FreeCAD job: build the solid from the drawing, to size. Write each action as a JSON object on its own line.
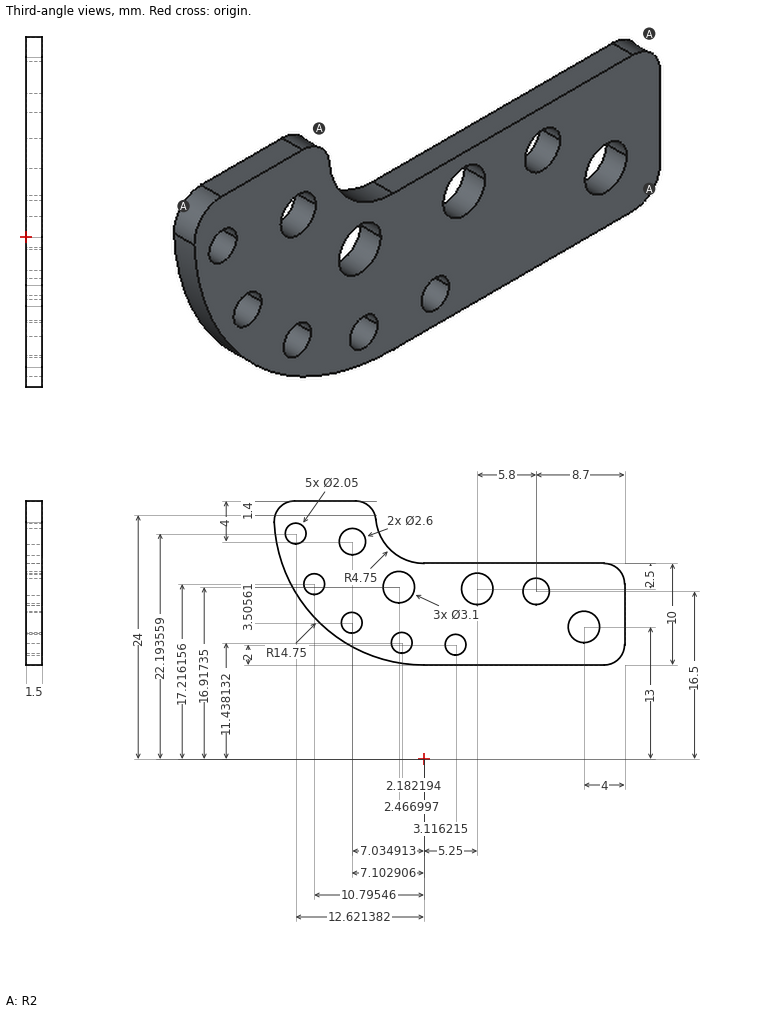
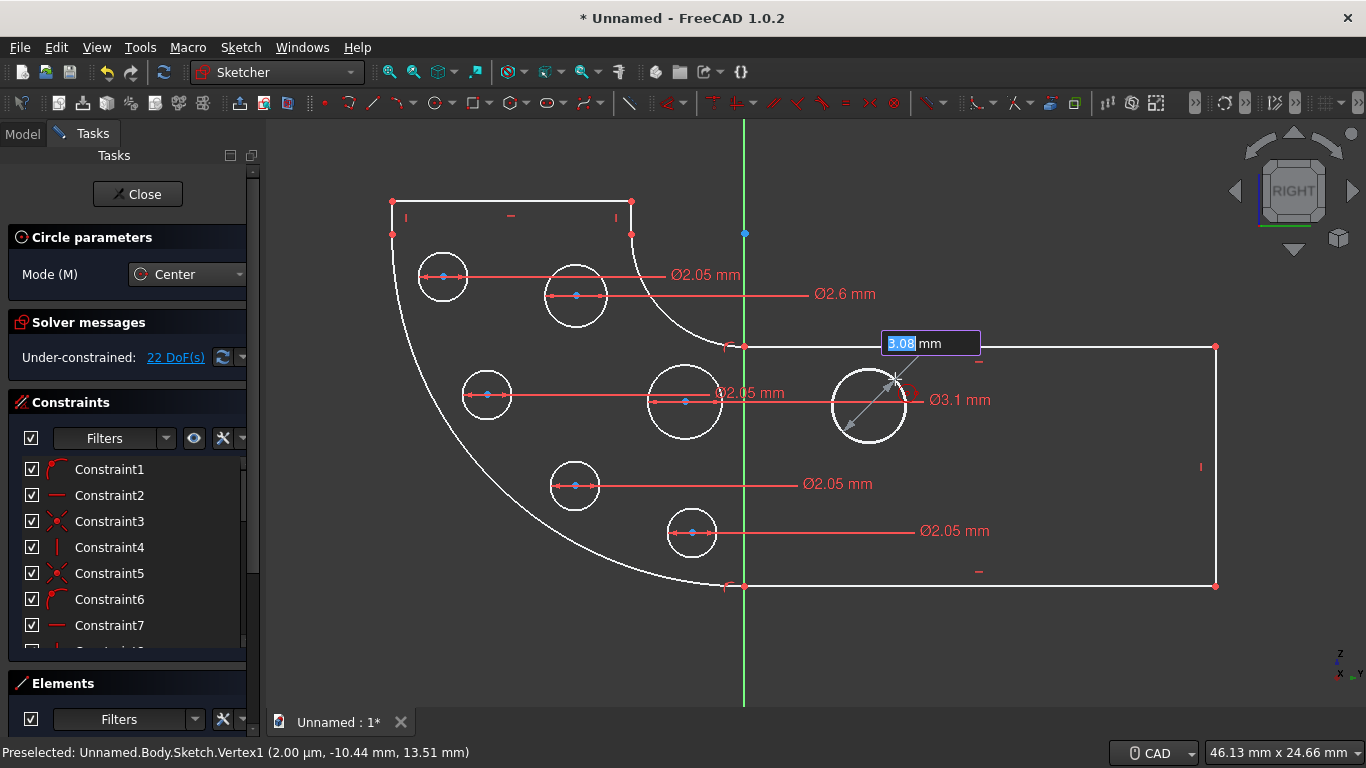
{"action": "type", "text": "3.1"}
{"action": "key", "text": "Return"}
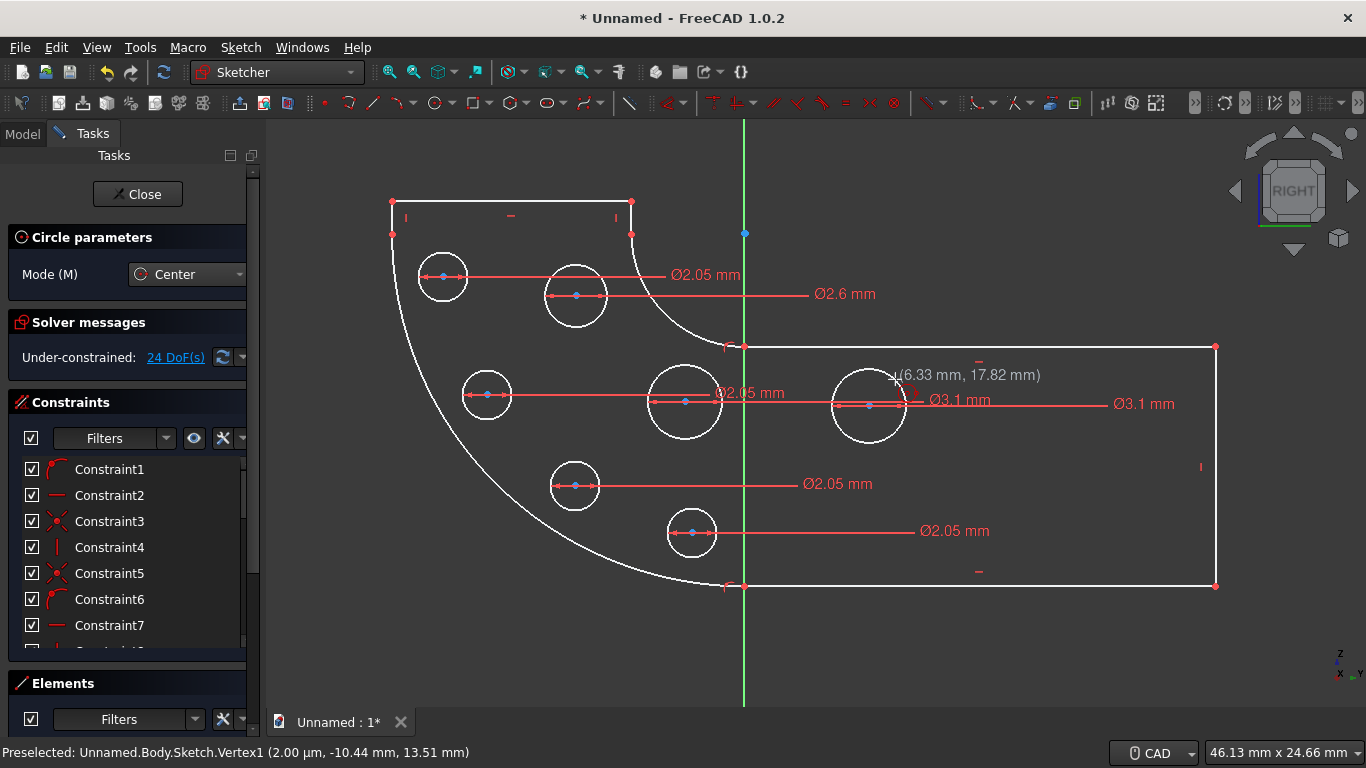
{"action": "left_click", "coordinate": [818, 537]}
{"action": "mouse_move", "coordinate": [836, 519]}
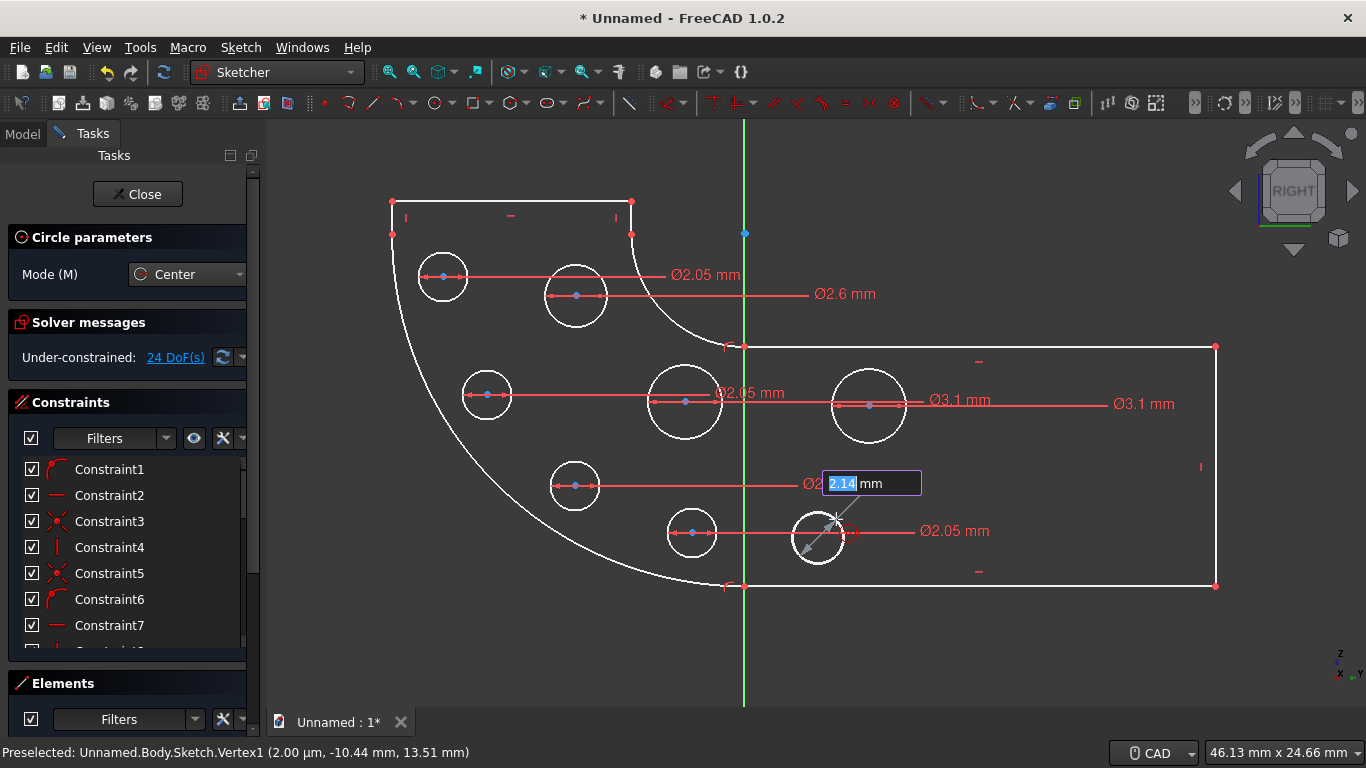
{"action": "type", "text": "2.05"}
{"action": "key", "text": "Return"}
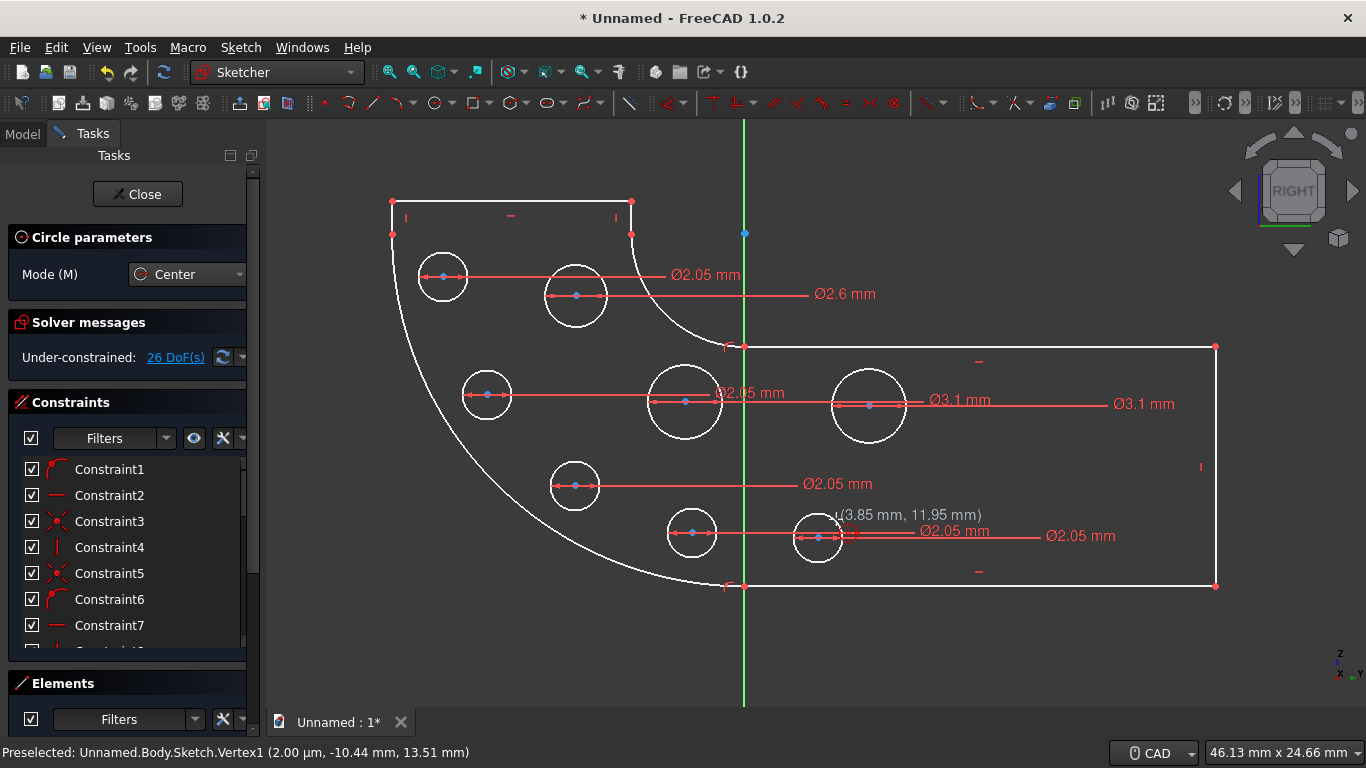
{"action": "left_click", "coordinate": [1008, 411]}
{"action": "mouse_move", "coordinate": [1030, 390]}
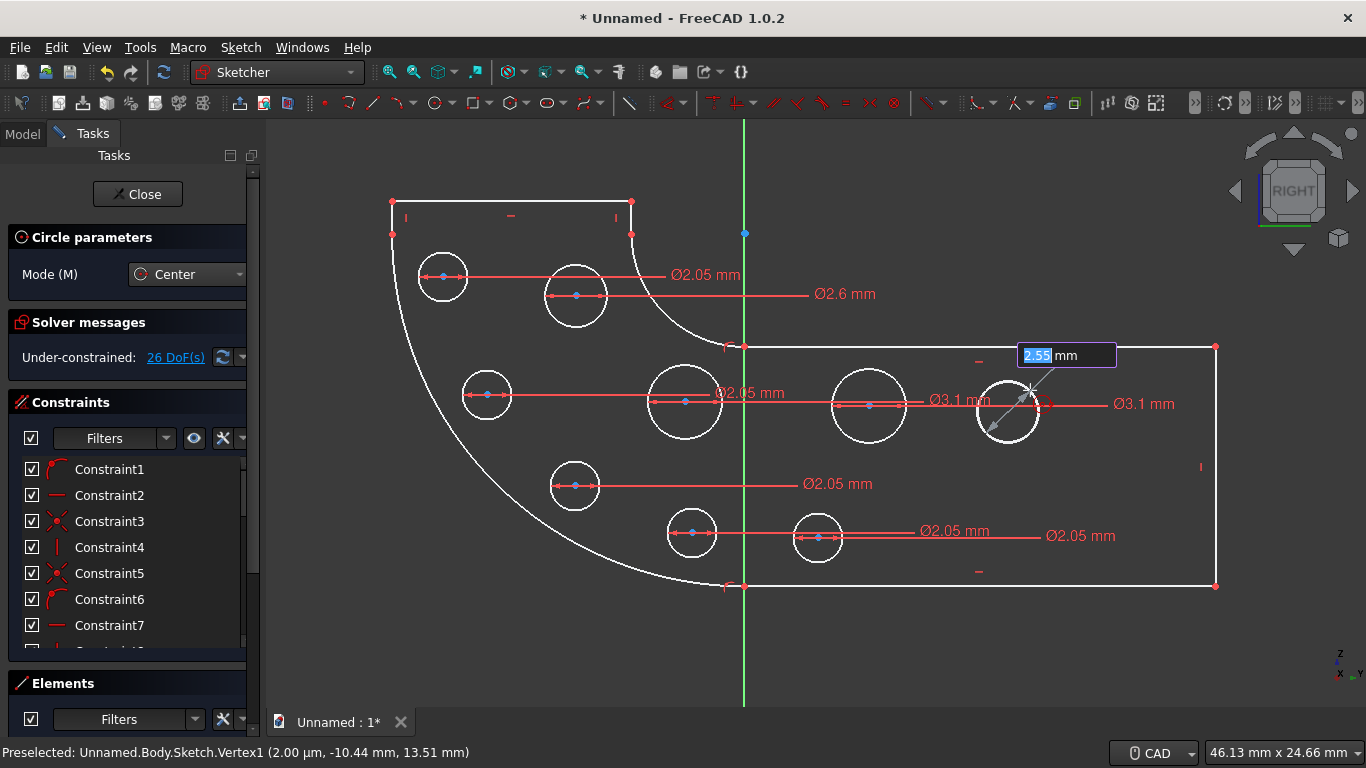
{"action": "type", "text": "2.6"}
{"action": "key", "text": "Return"}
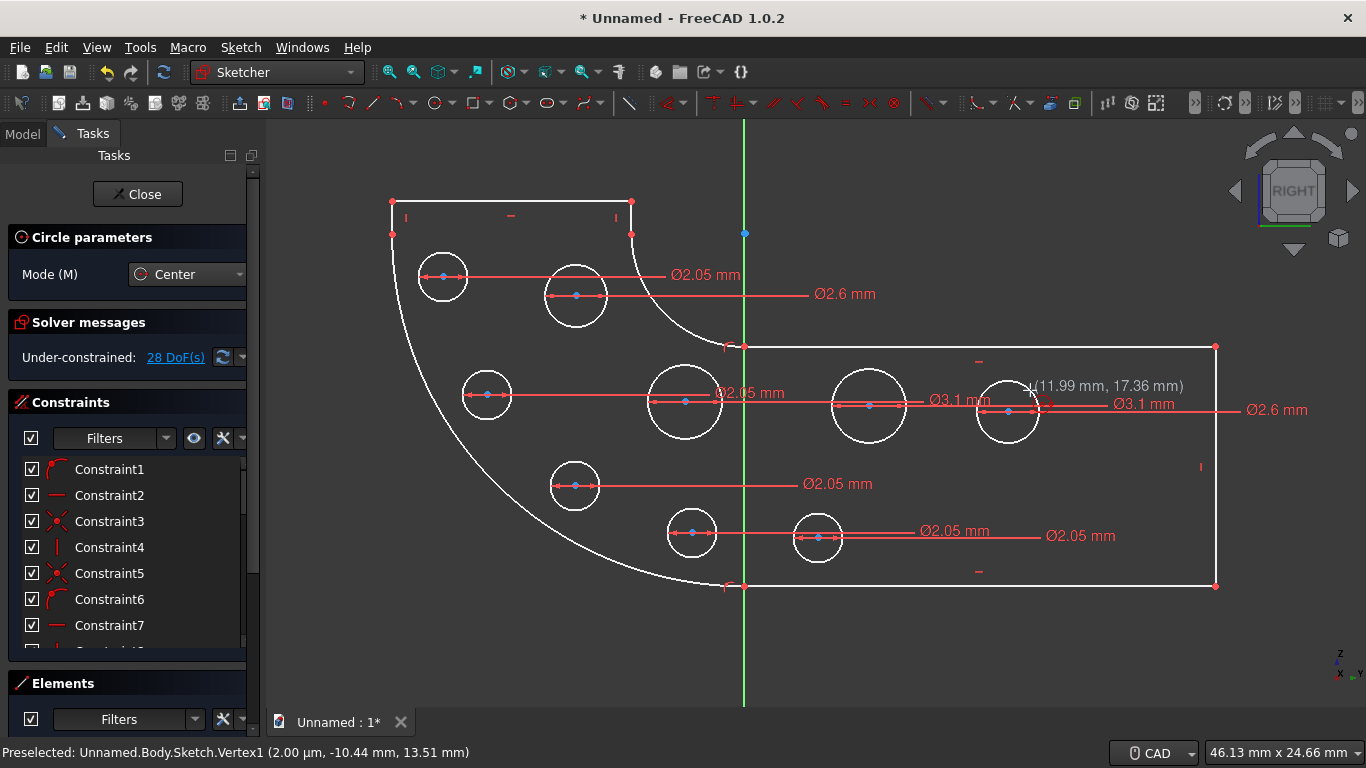
{"action": "left_click", "coordinate": [1120, 495]}
{"action": "mouse_move", "coordinate": [1146, 469]}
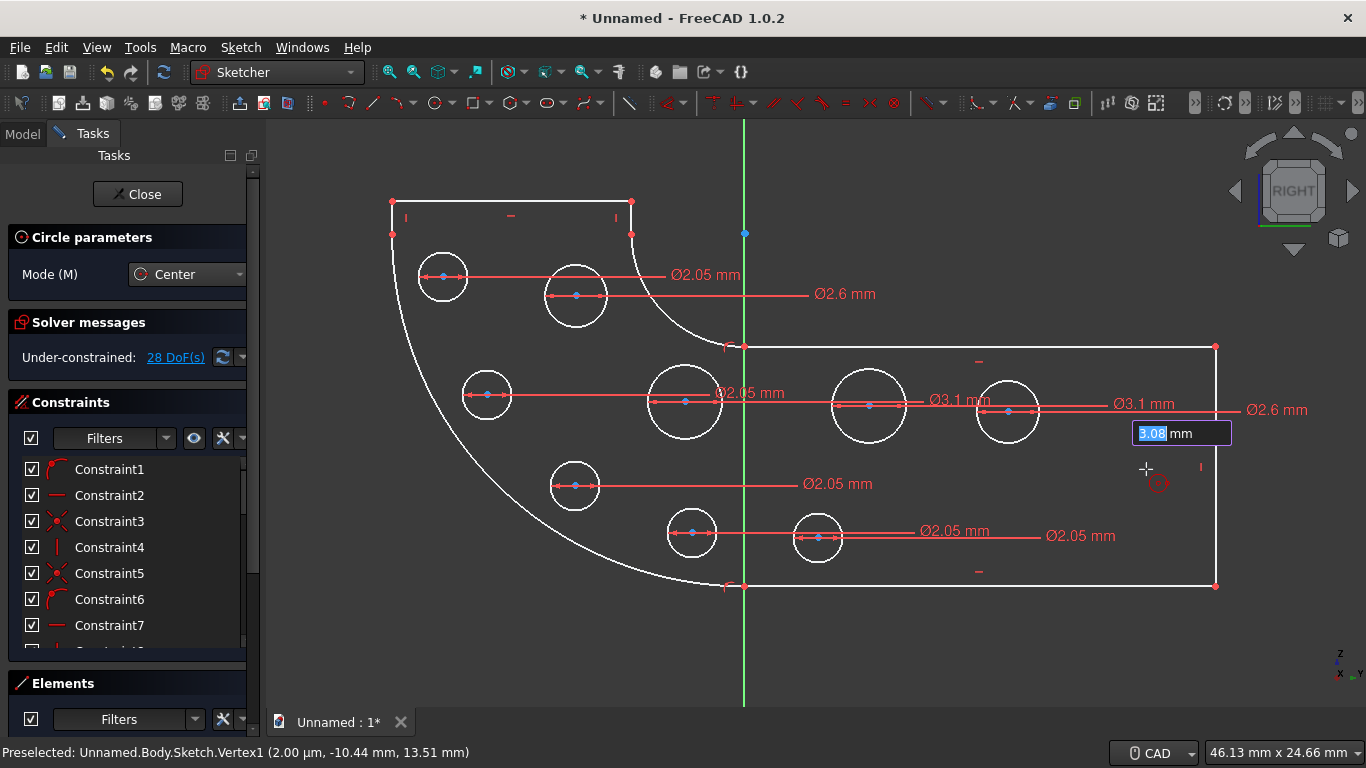
{"action": "type", "text": "3.1"}
{"action": "key", "text": "Return"}
{"action": "key", "text": "Escape"}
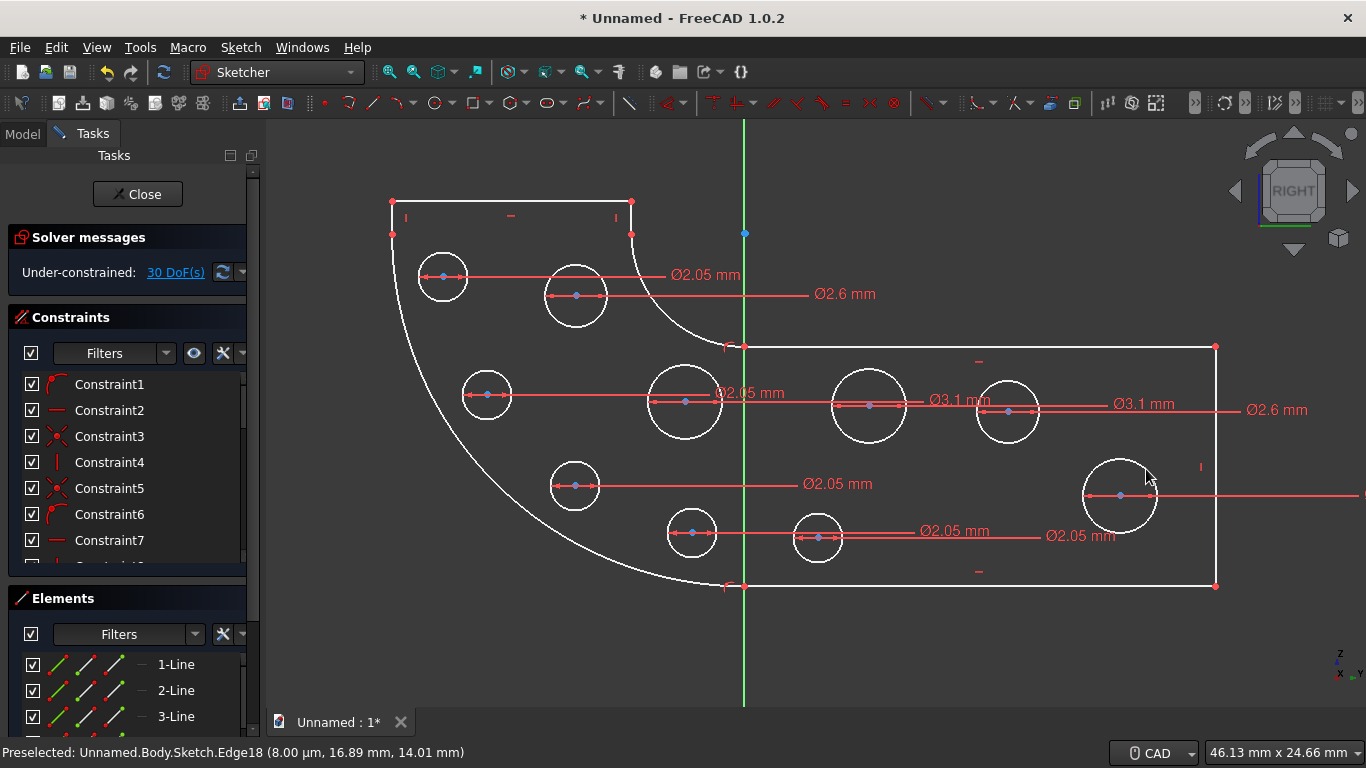
{"action": "left_click", "coordinate": [886, 586]}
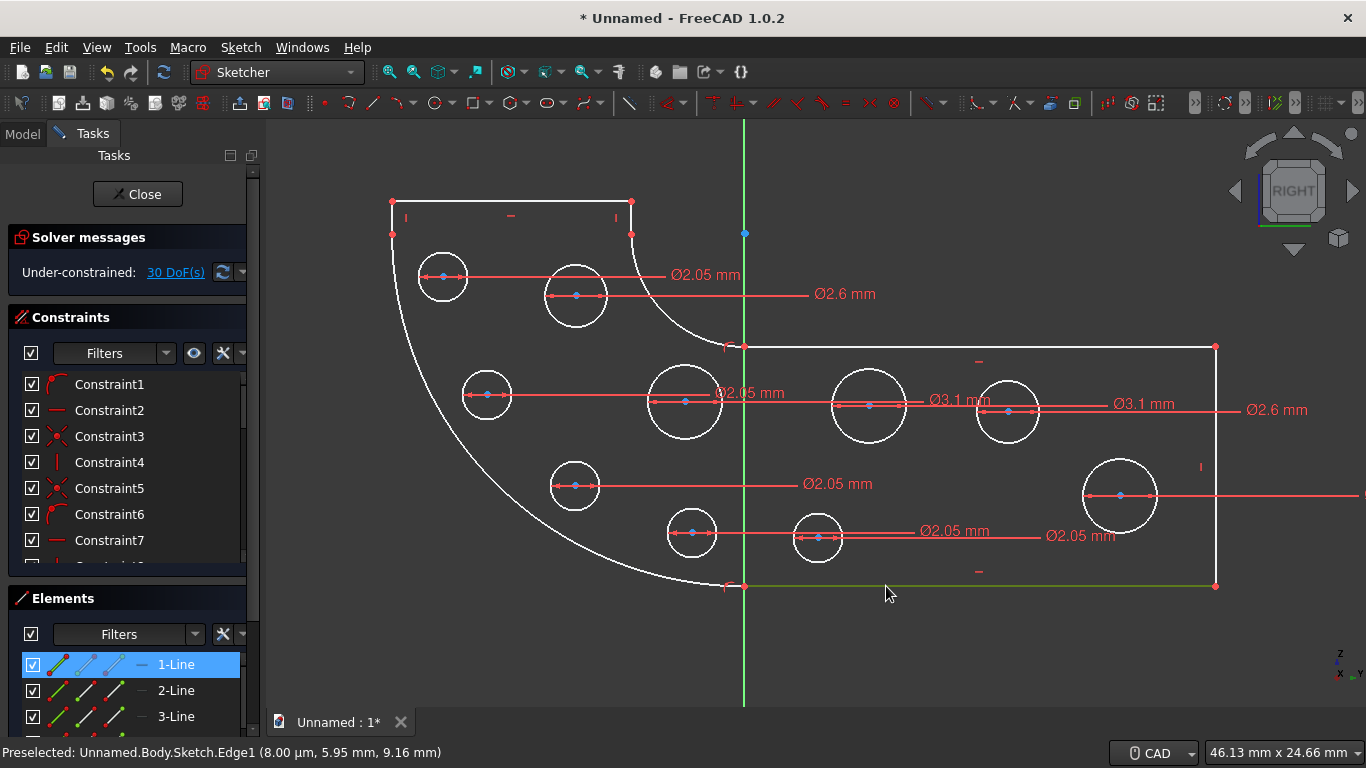
{"action": "left_click", "coordinate": [431, 394]}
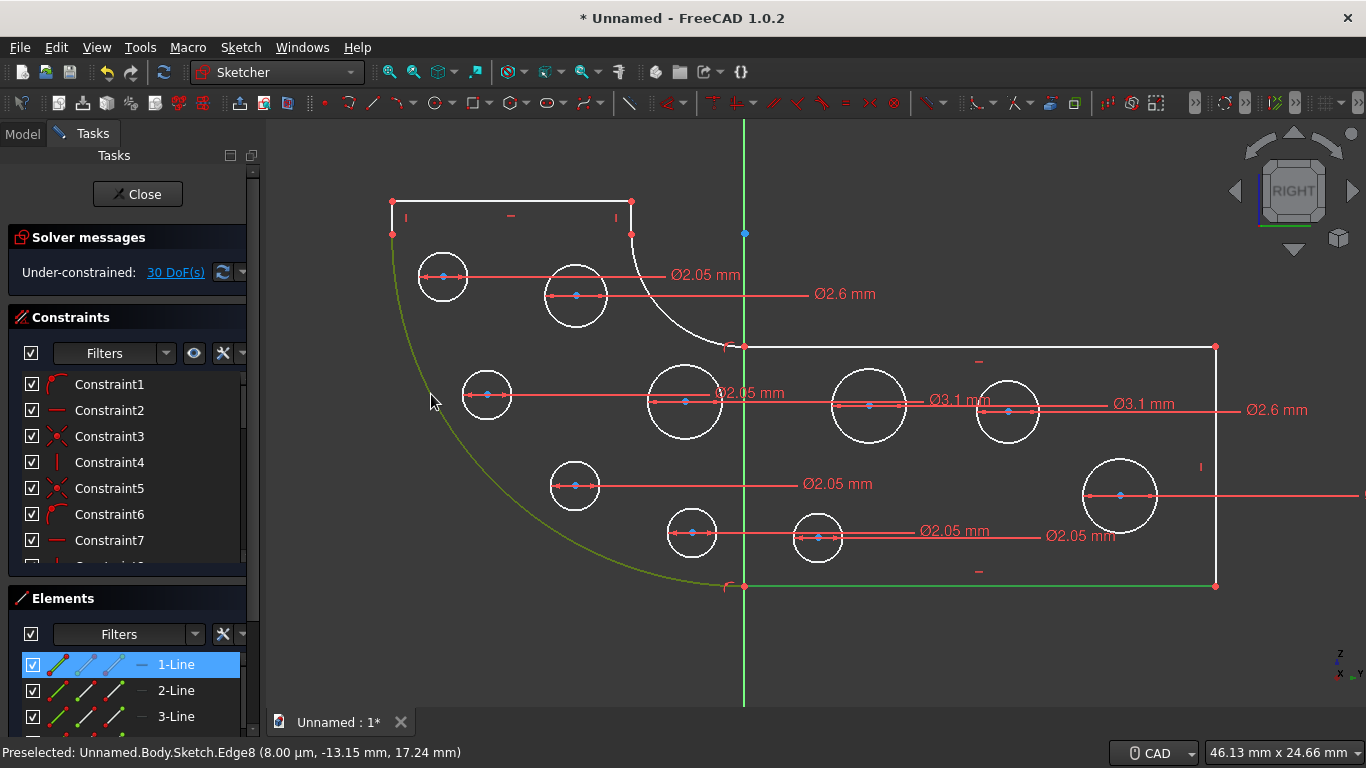
{"action": "left_click", "coordinate": [822, 104]}